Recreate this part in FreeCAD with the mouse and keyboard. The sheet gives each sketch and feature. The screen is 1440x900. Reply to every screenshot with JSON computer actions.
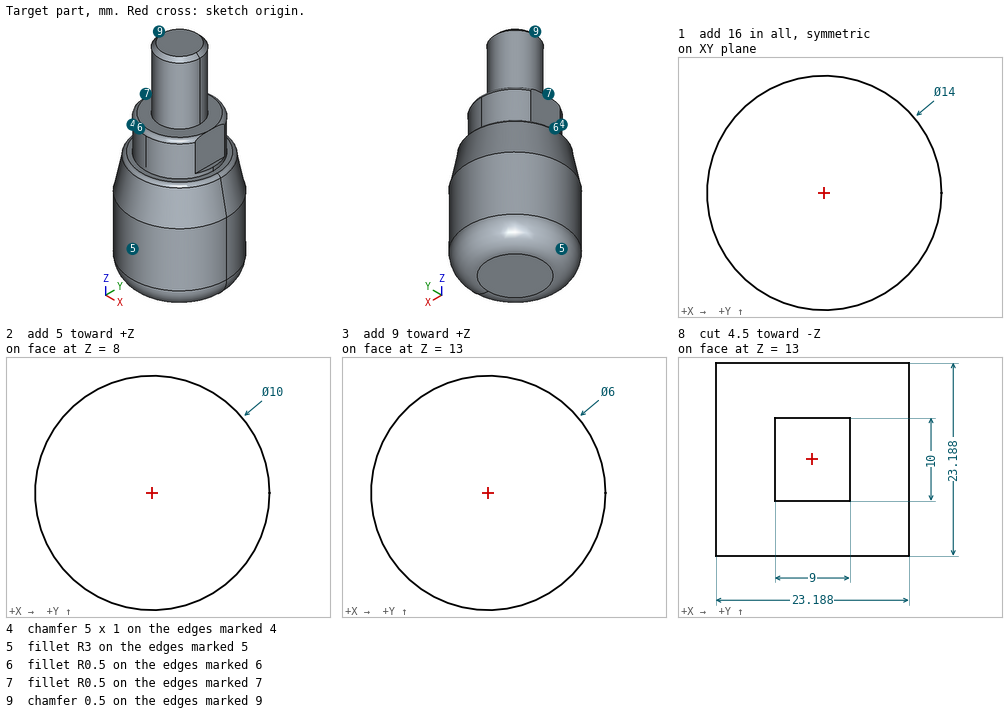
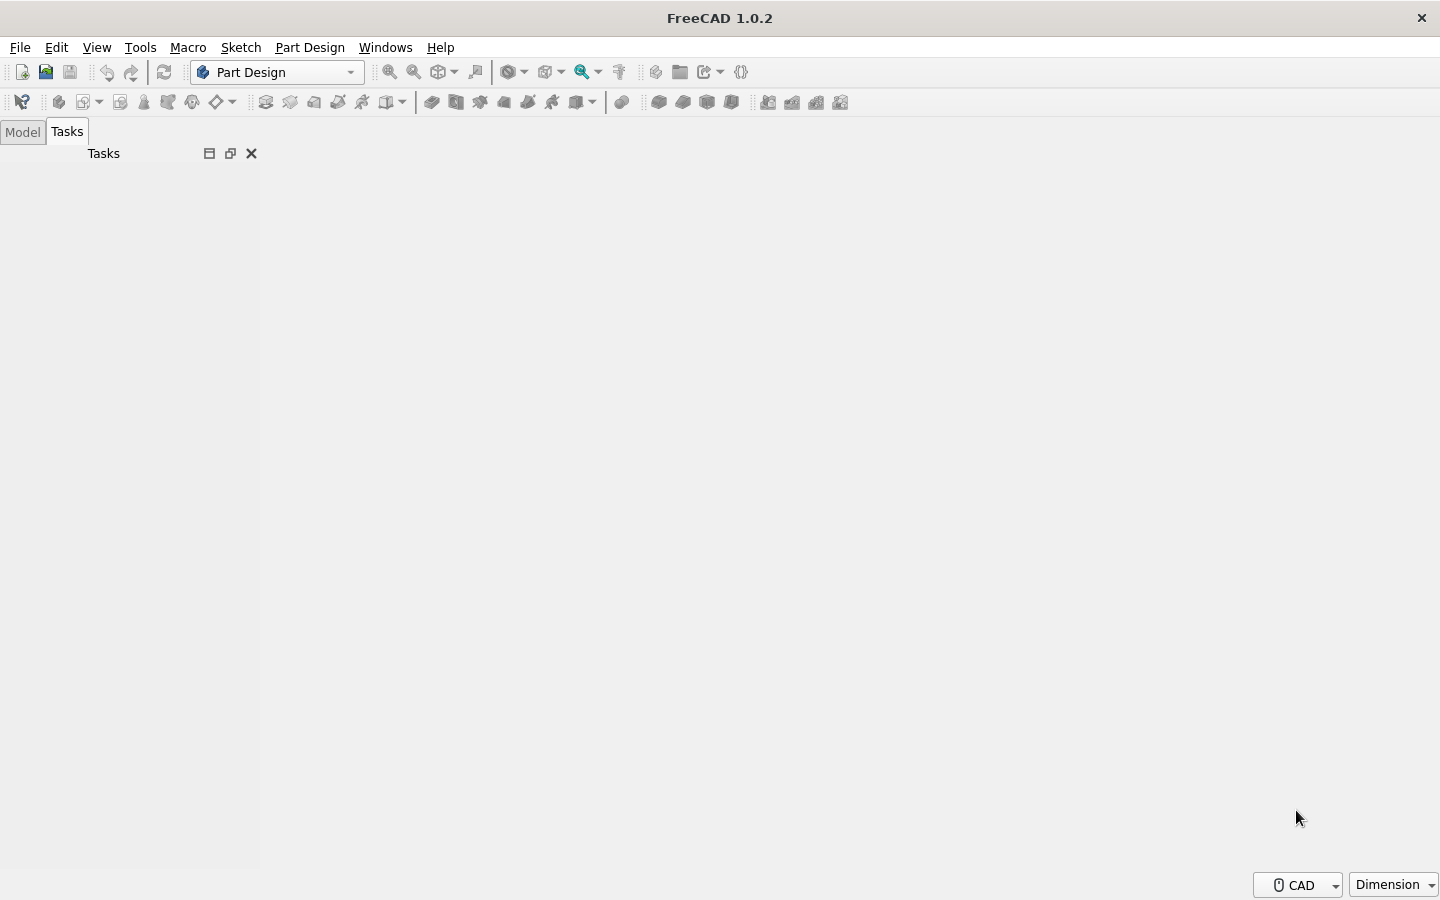
{"action": "key", "text": "ctrl+n"}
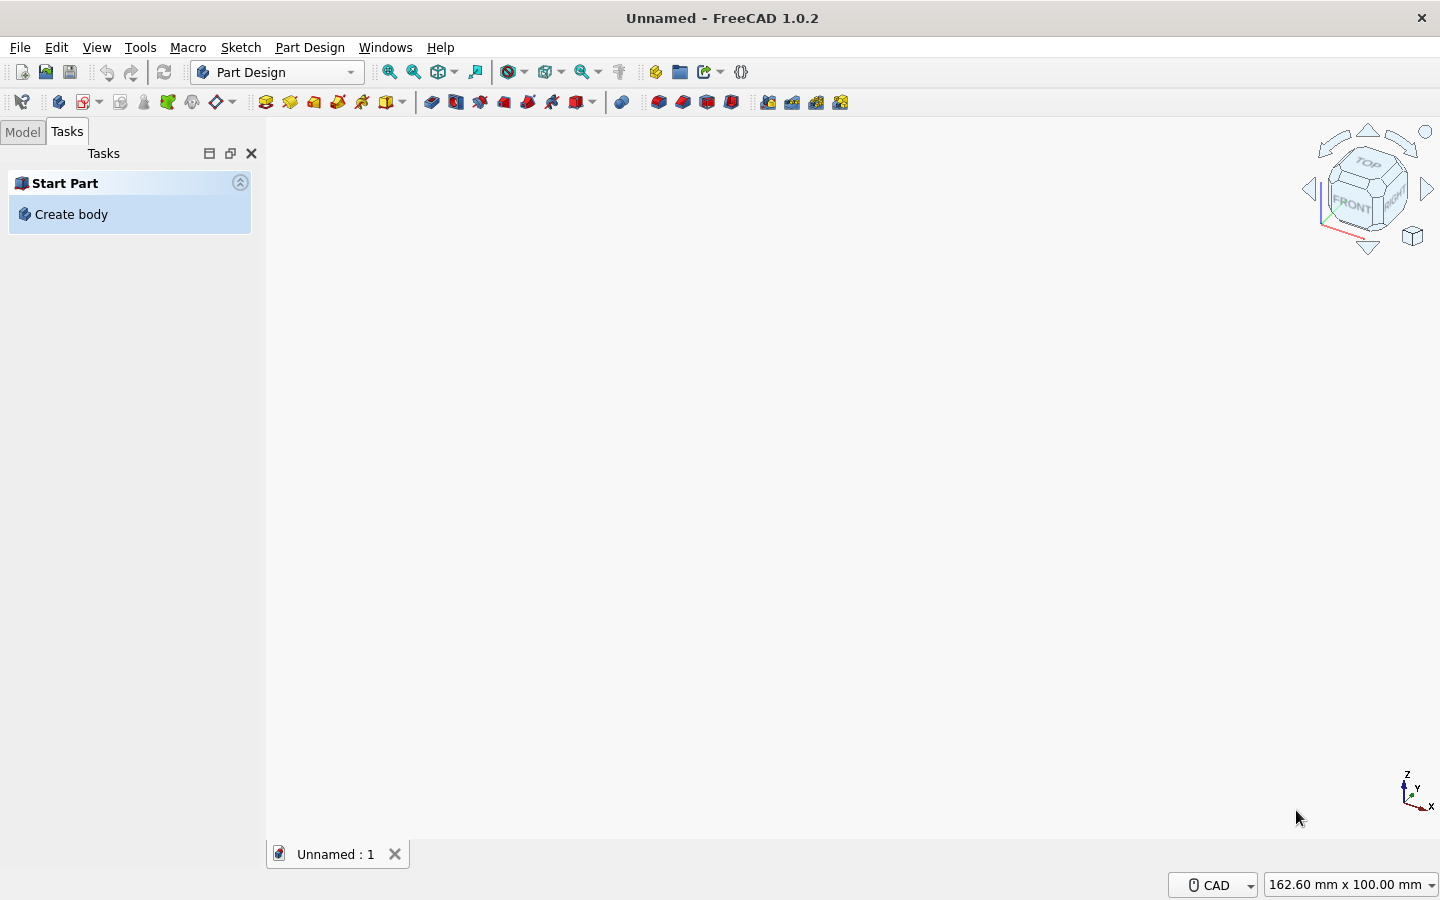
{"action": "left_click", "coordinate": [84, 102]}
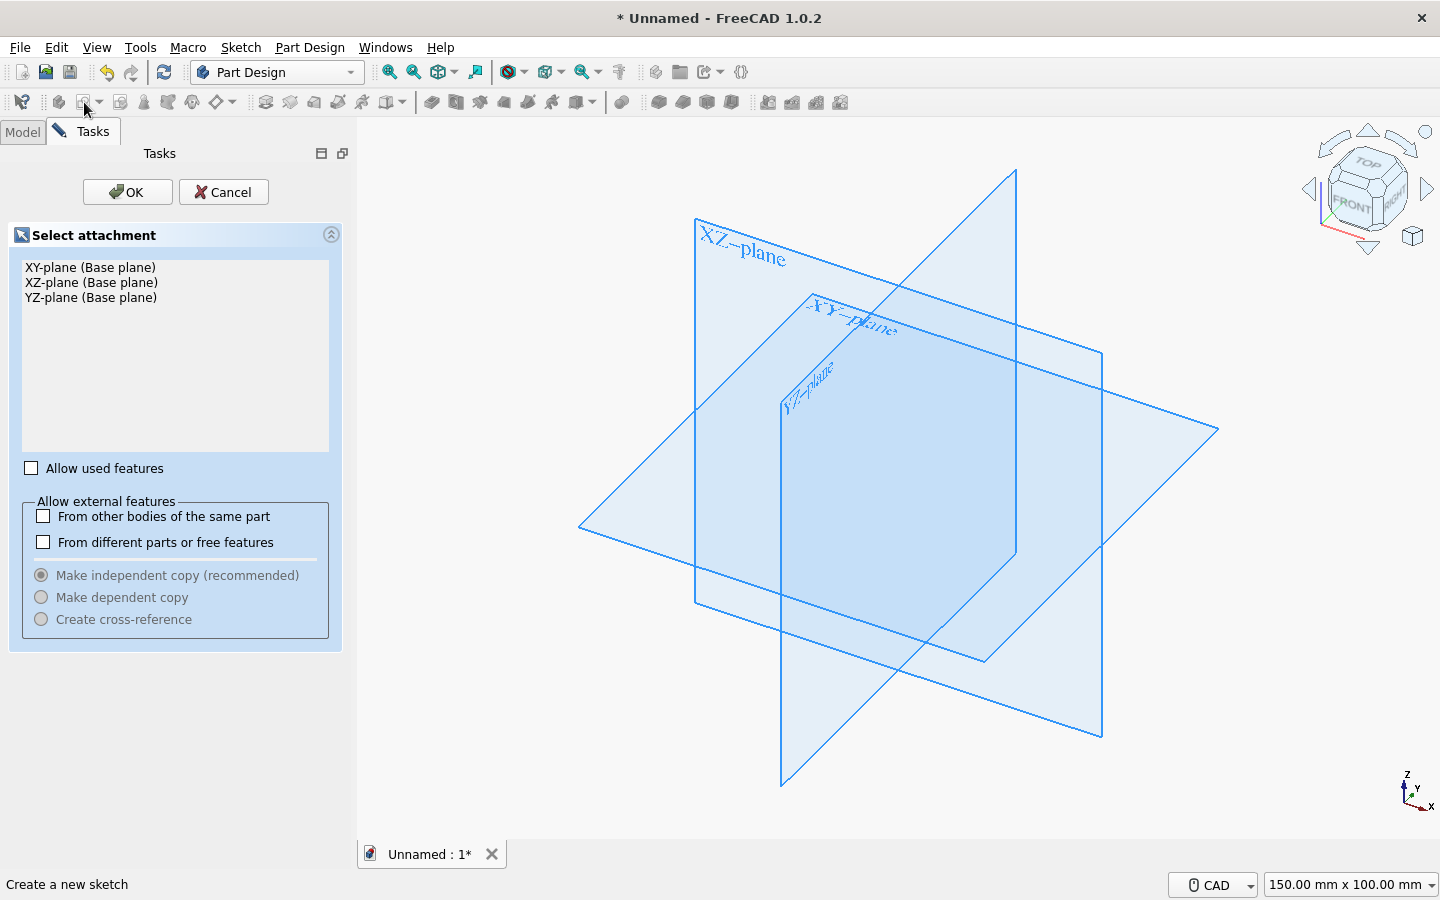
{"action": "left_click", "coordinate": [82, 268]}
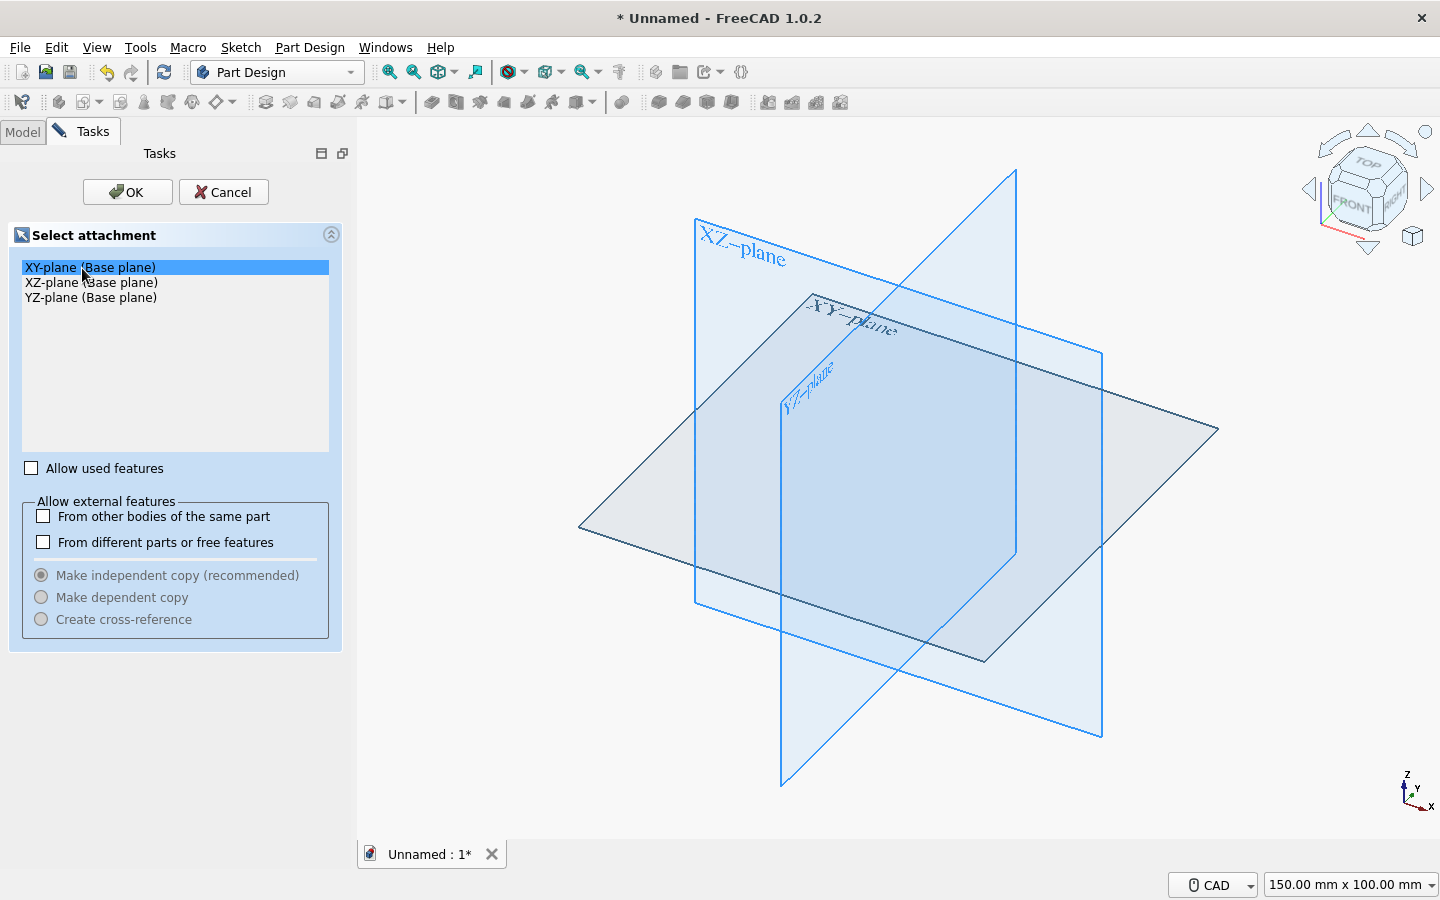
{"action": "left_click", "coordinate": [128, 192]}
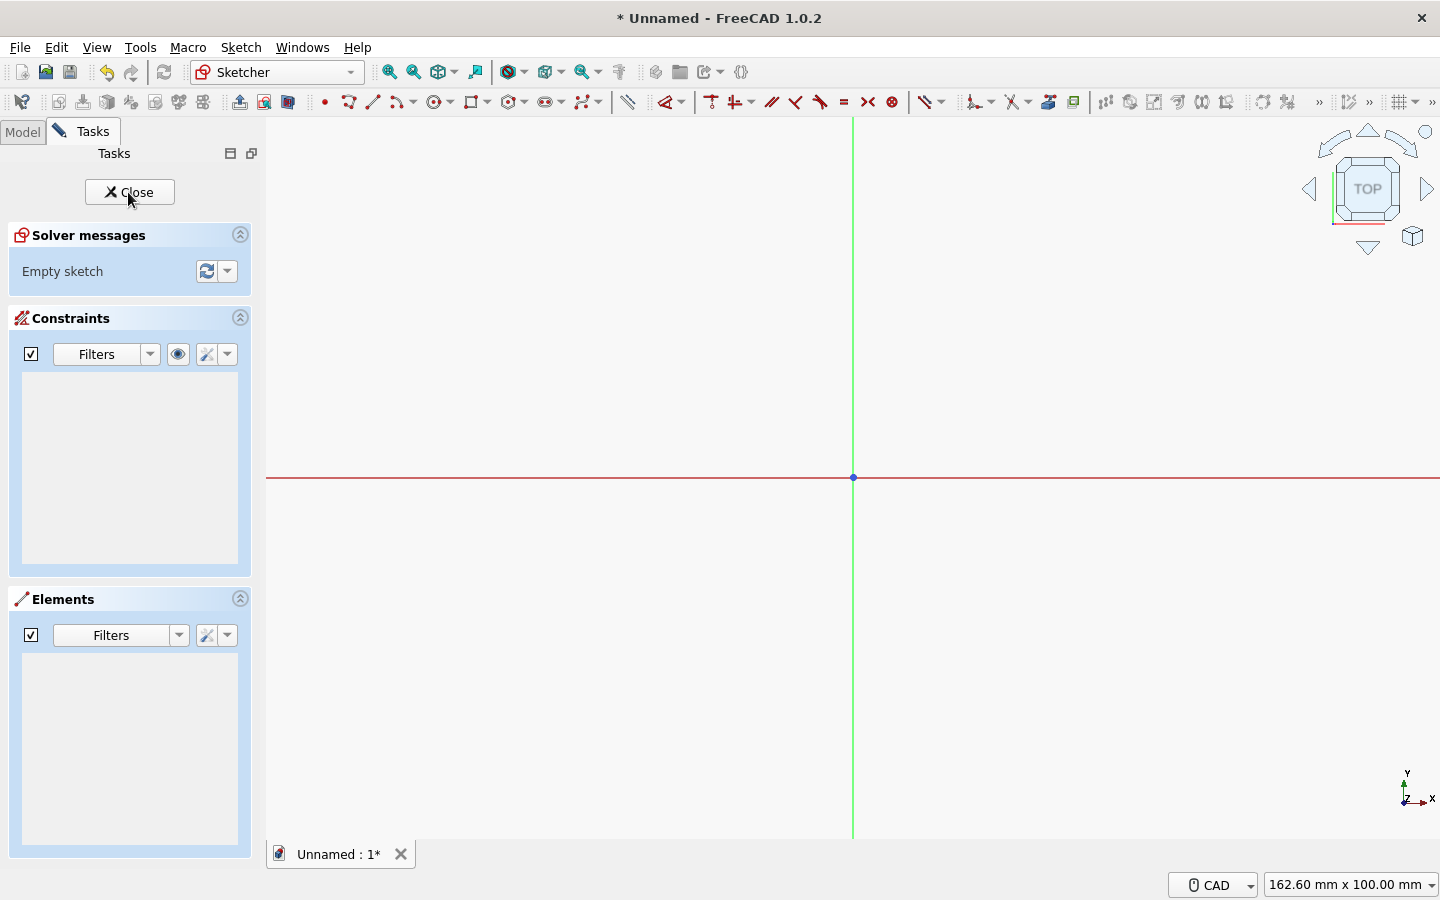
{"action": "scroll", "coordinate": [870, 478], "scroll_direction": "up", "scroll_amount": 8}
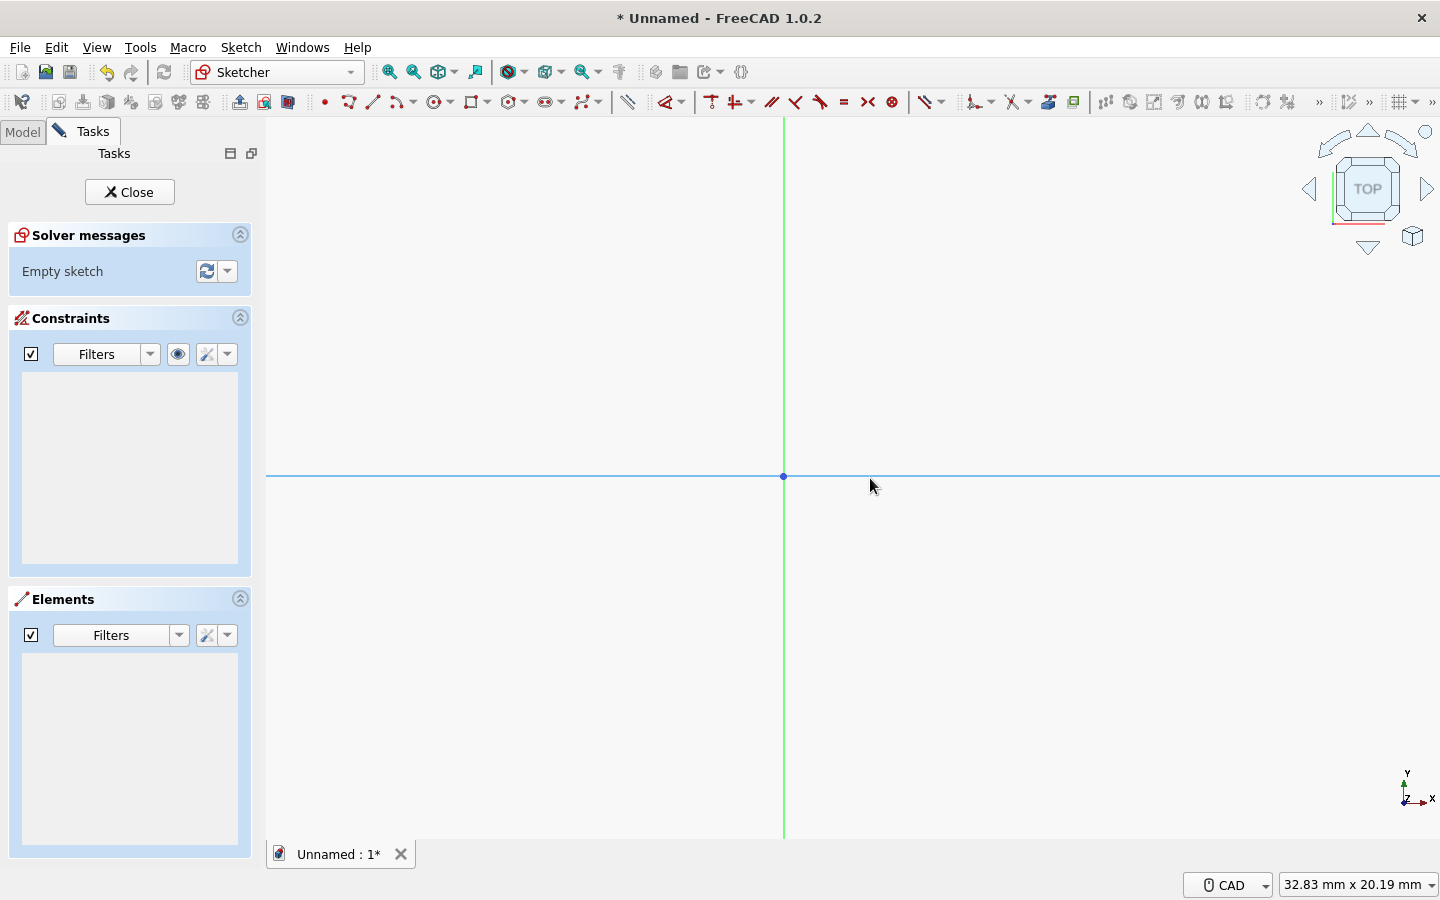
{"action": "left_click", "coordinate": [434, 102]}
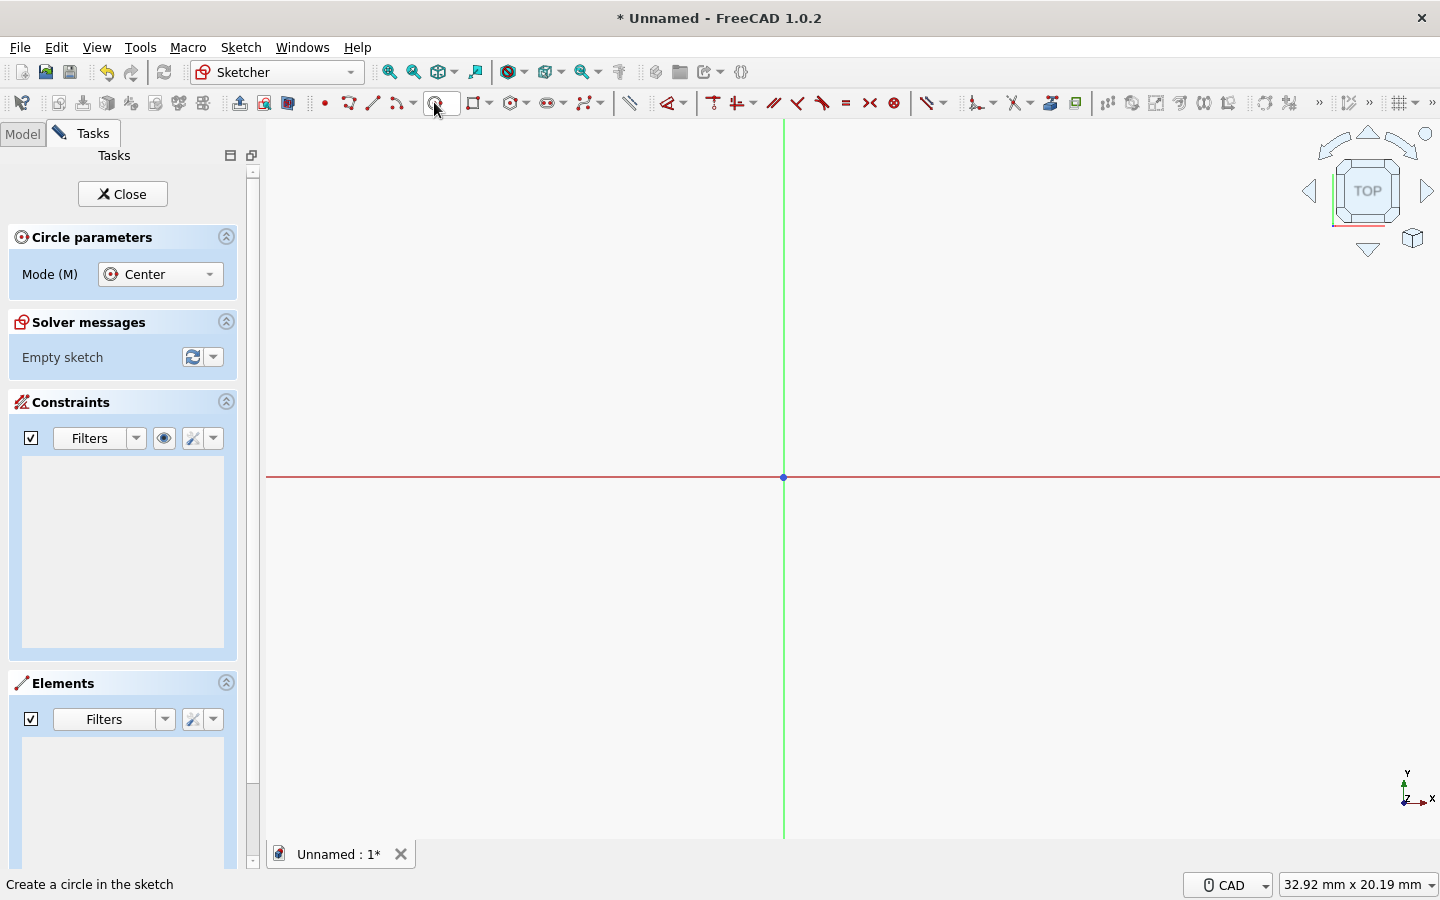
{"action": "left_click", "coordinate": [784, 477]}
{"action": "left_click", "coordinate": [960, 301]}
{"action": "key", "text": "Escape"}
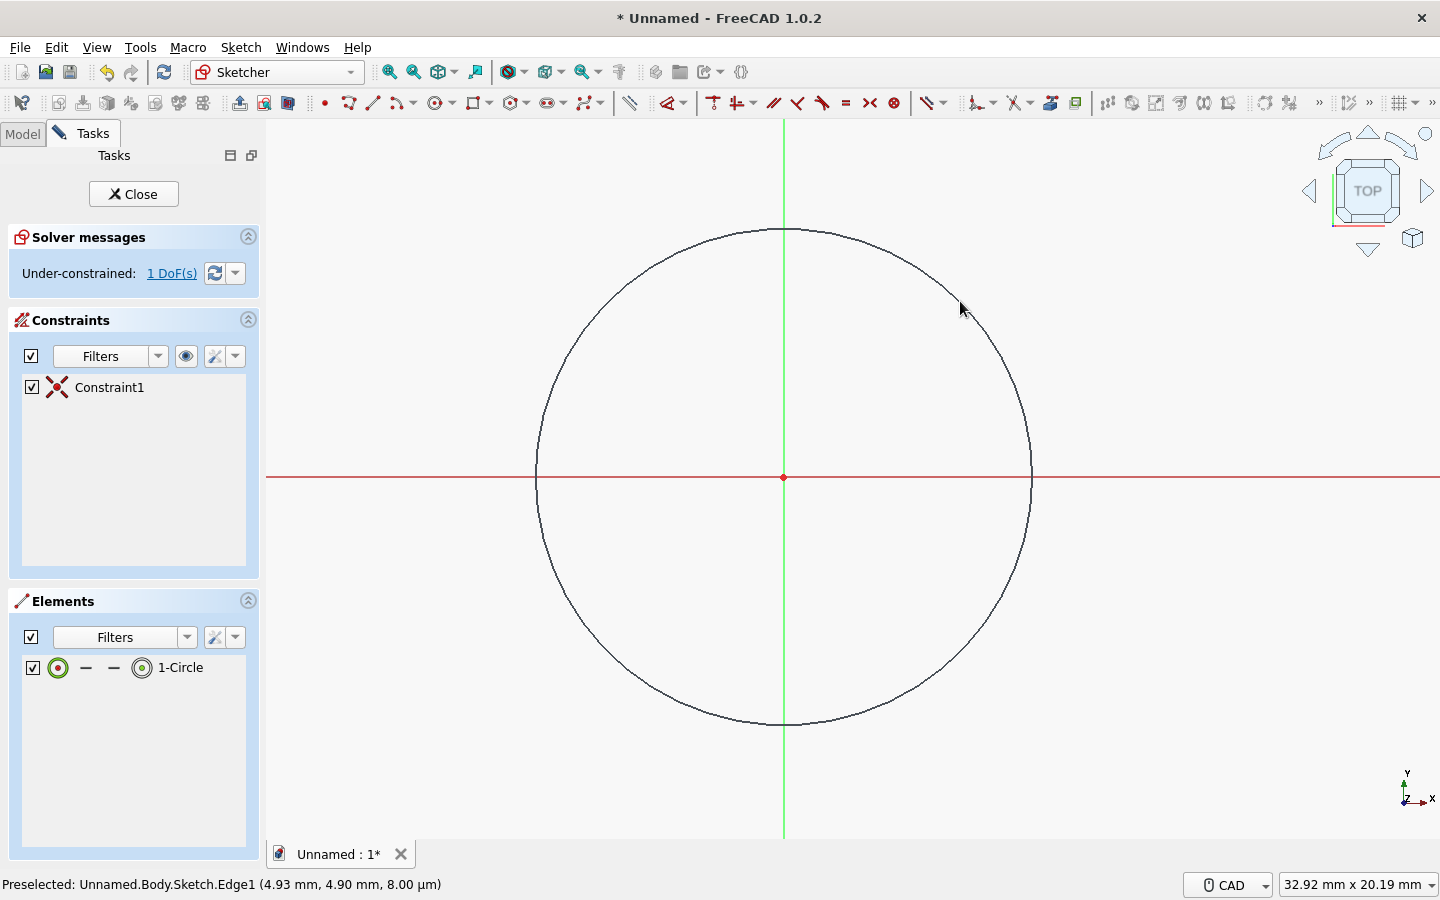
{"action": "left_click", "coordinate": [959, 301]}